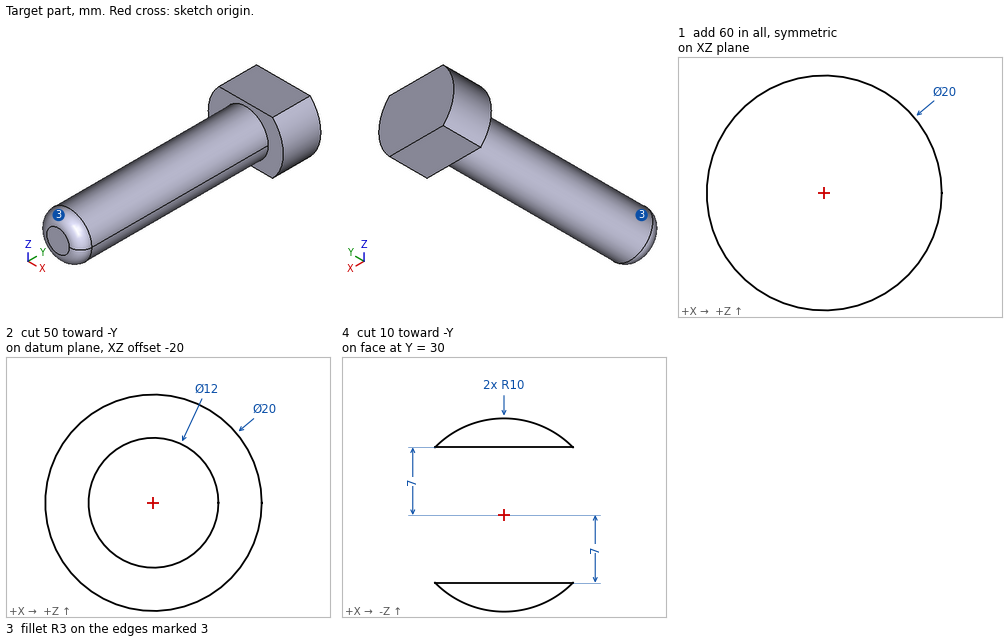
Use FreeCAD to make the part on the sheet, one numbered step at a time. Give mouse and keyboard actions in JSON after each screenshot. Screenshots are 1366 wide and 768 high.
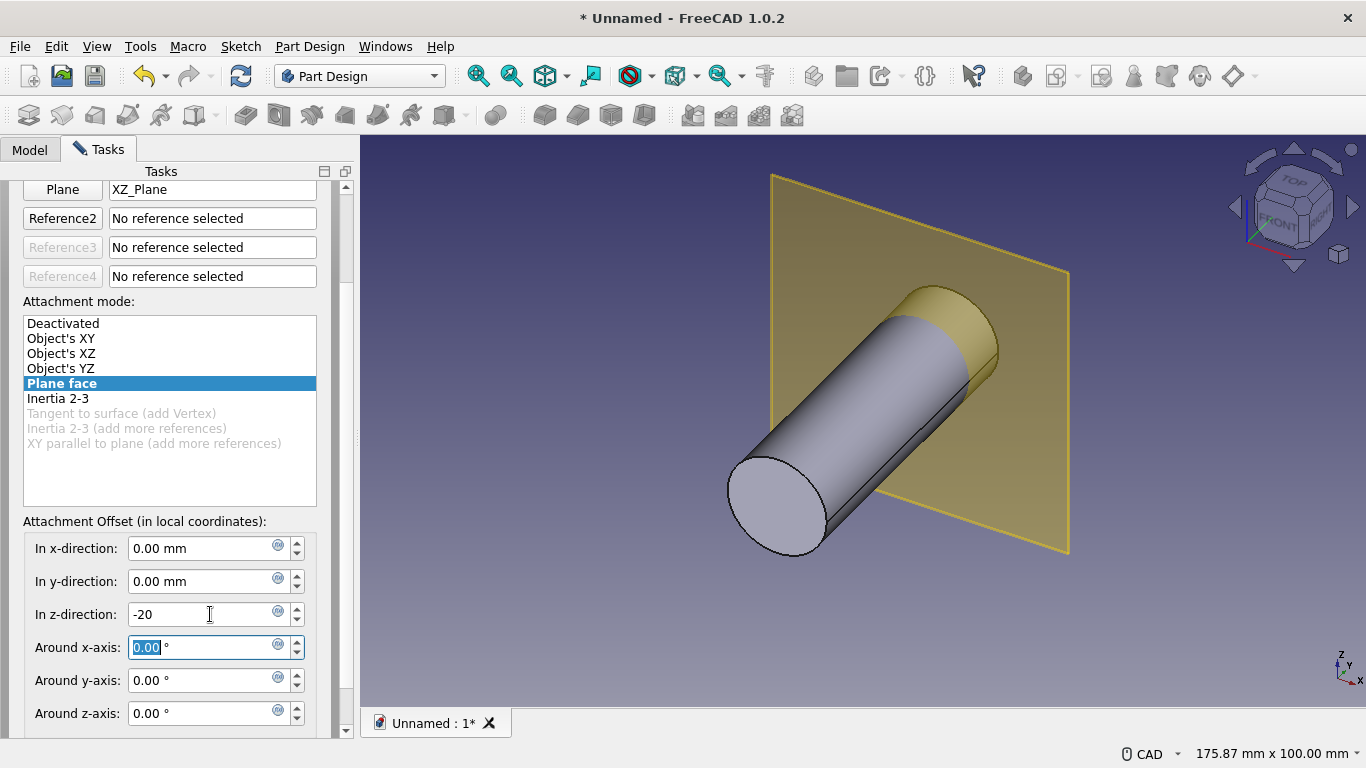
{"action": "scroll", "coordinate": [346, 460], "scroll_direction": "up", "scroll_amount": 3}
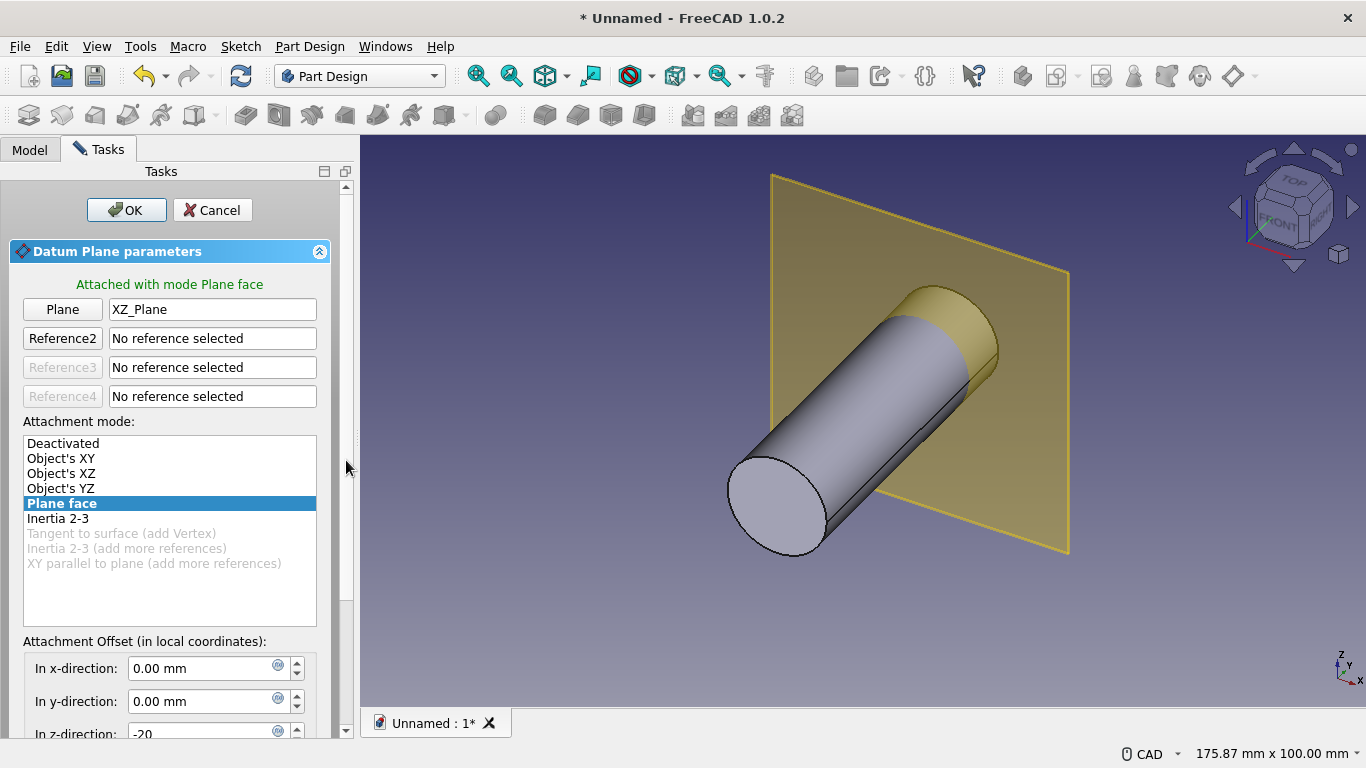
{"action": "left_click", "coordinate": [127, 210]}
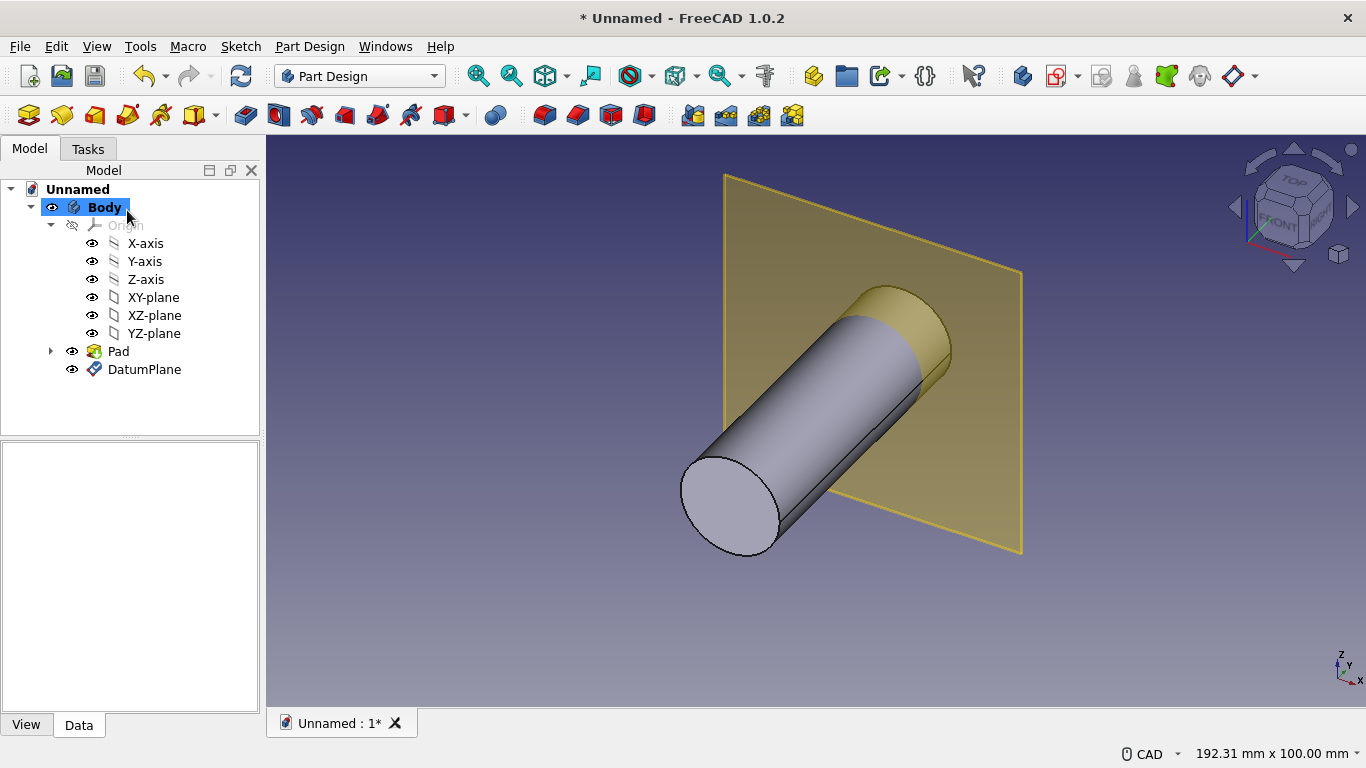
{"action": "left_click", "coordinate": [117, 369]}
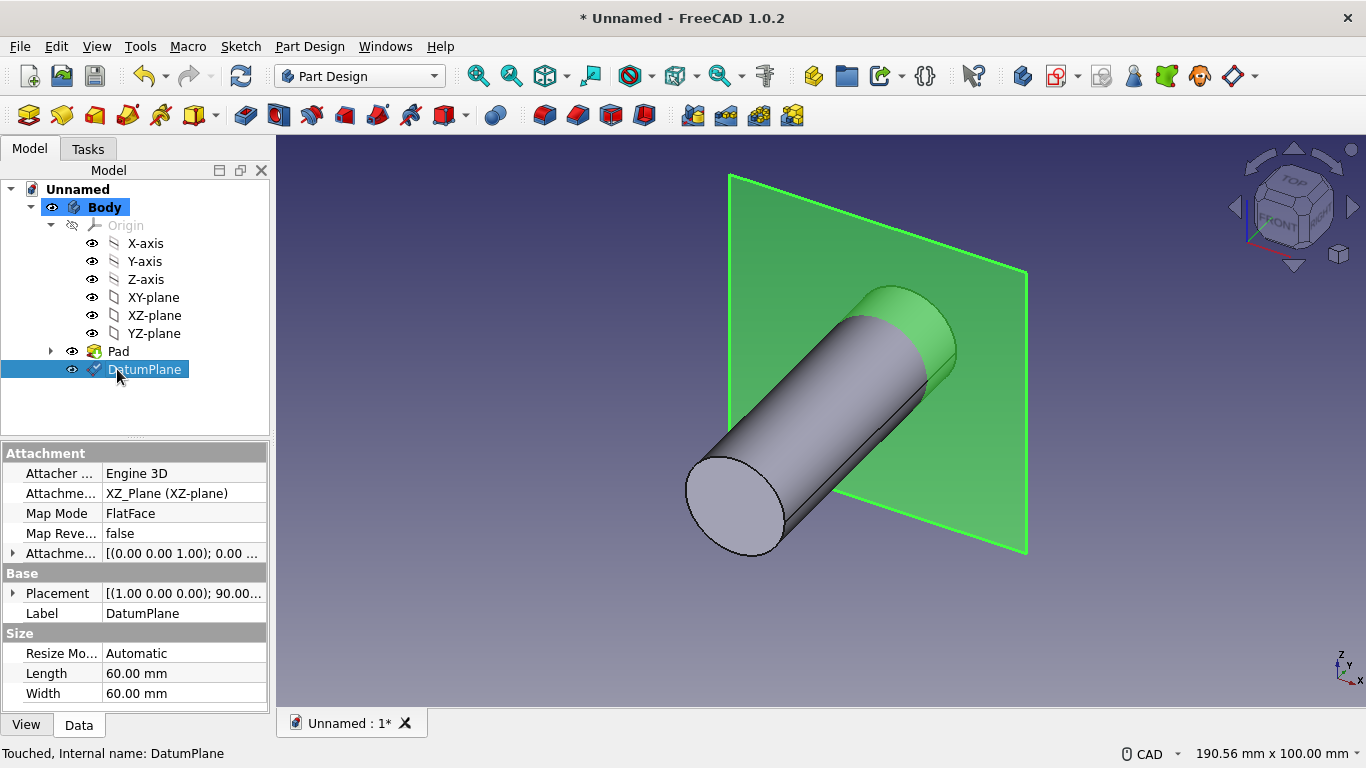
{"action": "left_click", "coordinate": [1056, 76]}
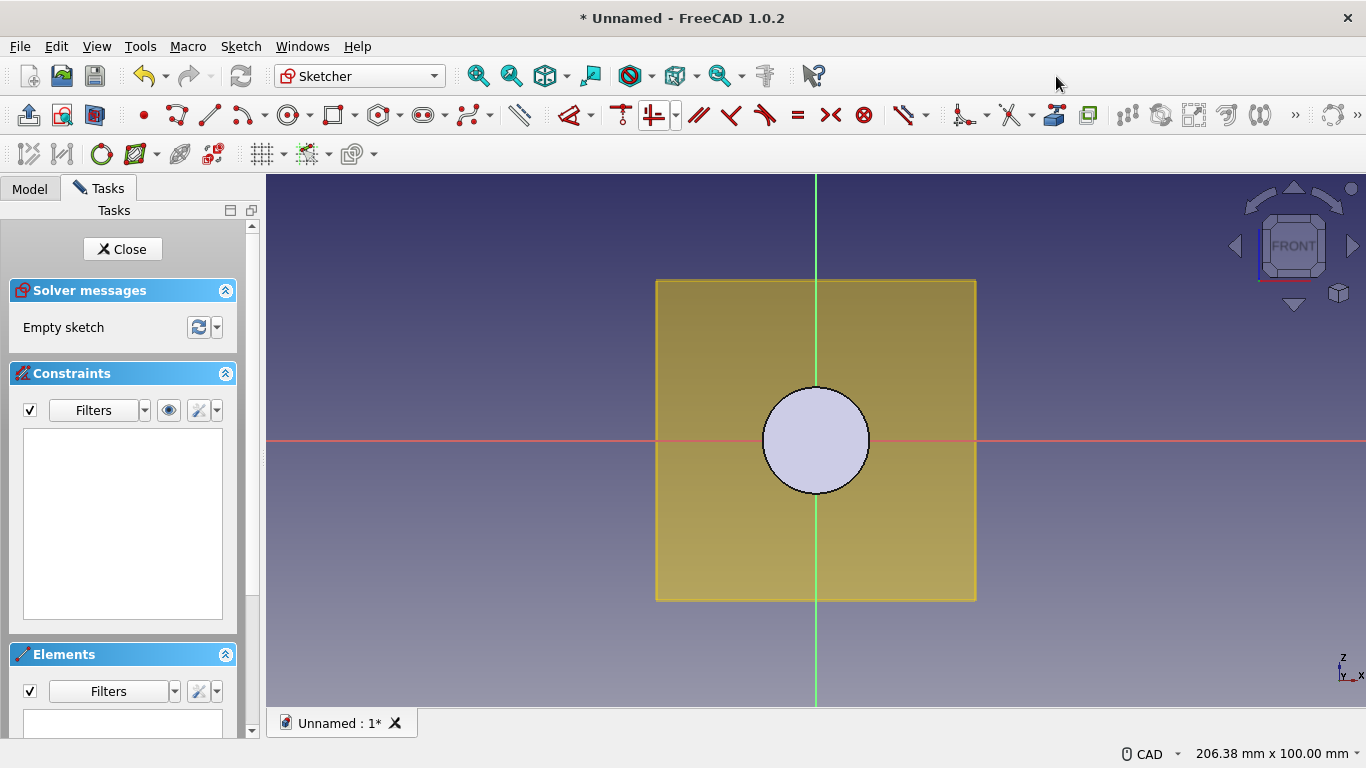
{"action": "left_click", "coordinate": [95, 116]}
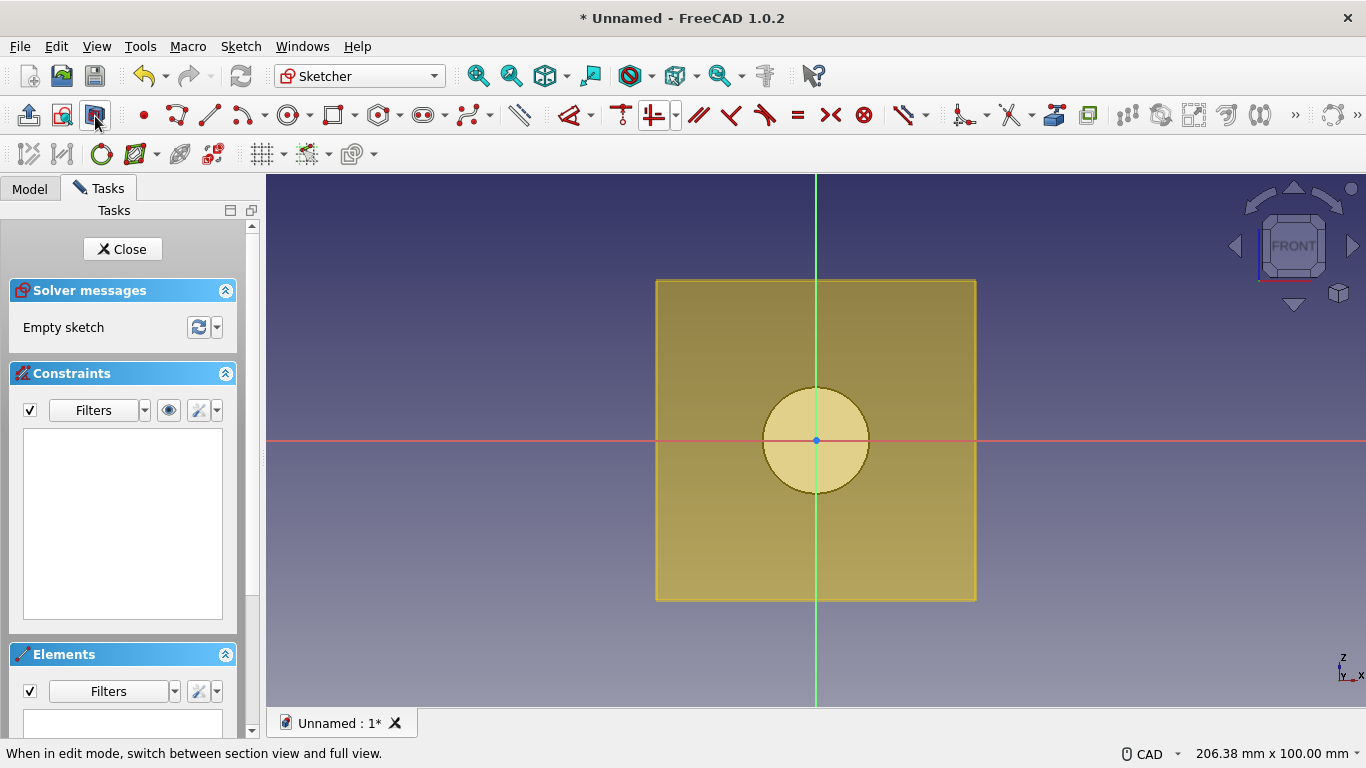
{"action": "scroll", "coordinate": [846, 440], "scroll_direction": "up", "scroll_amount": 6}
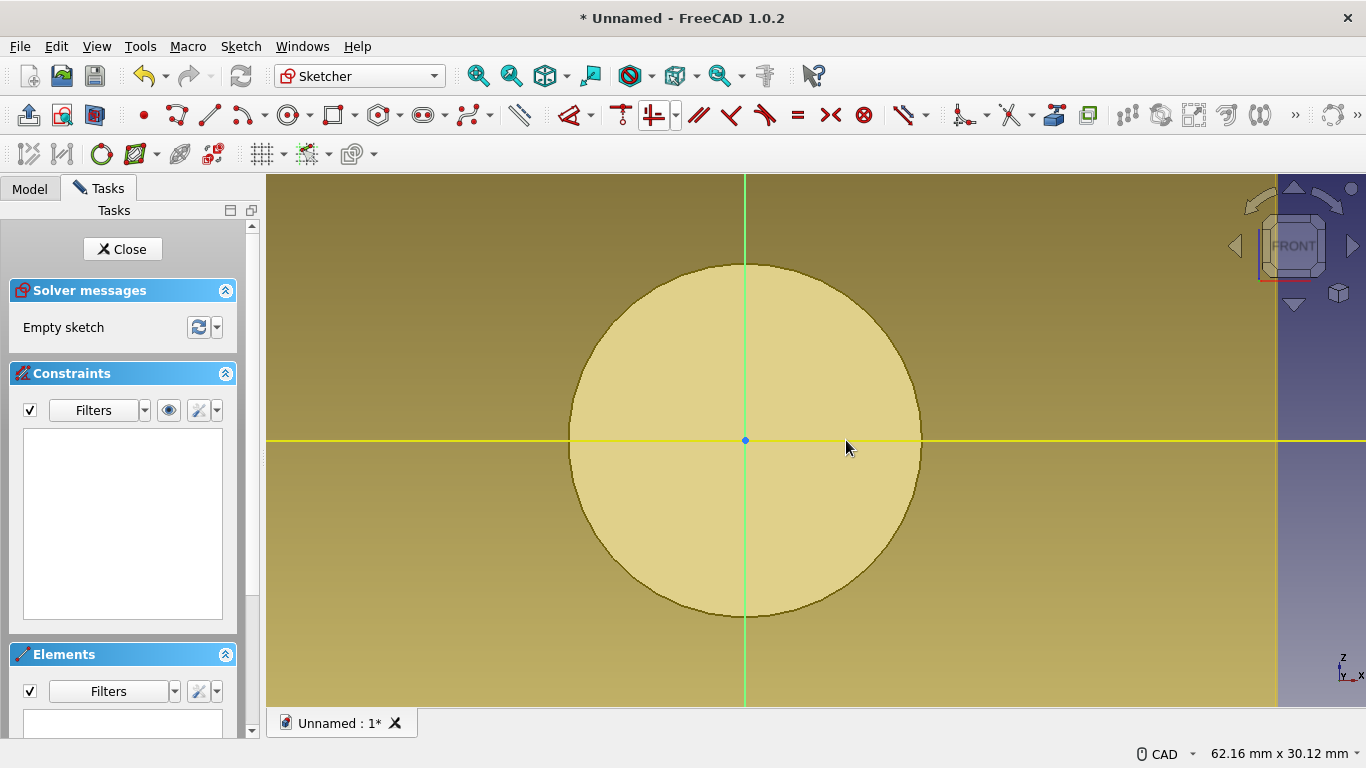
{"action": "left_click", "coordinate": [288, 116]}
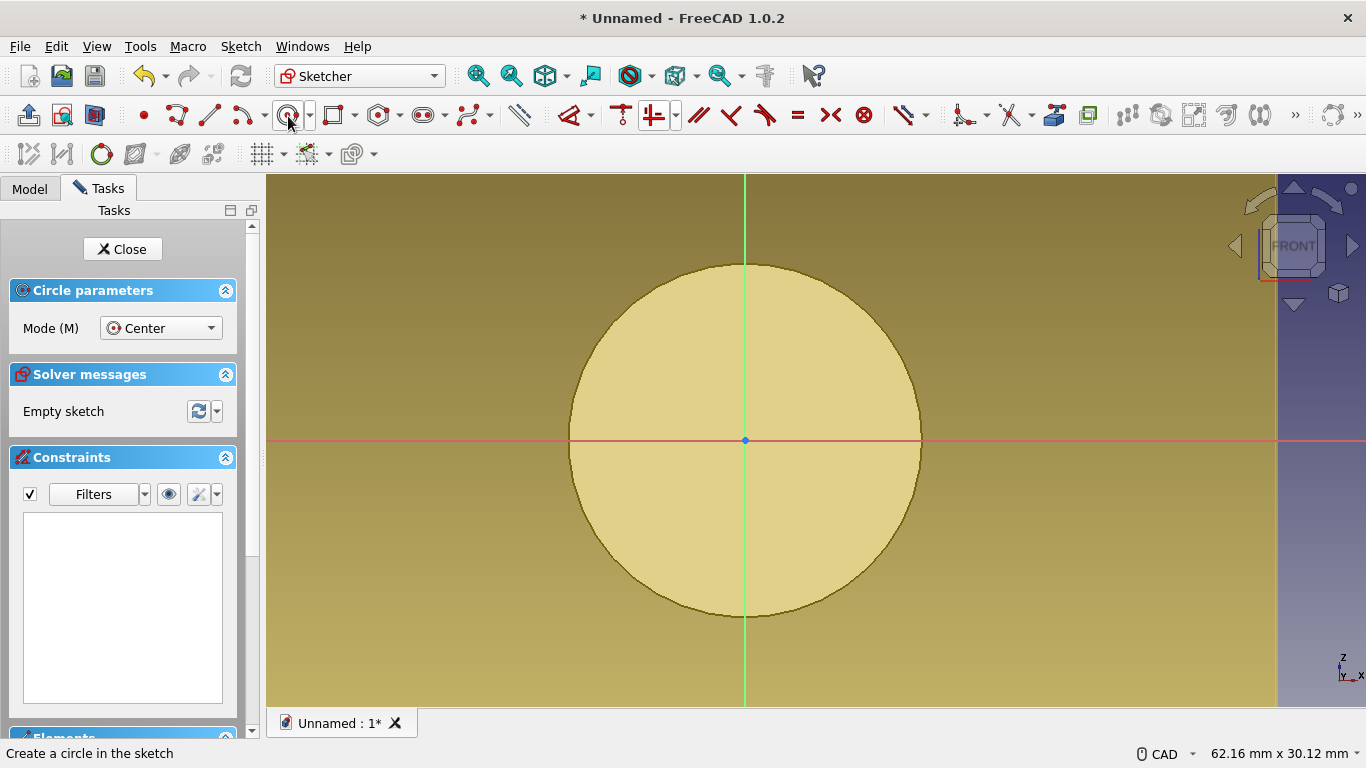
{"action": "left_click", "coordinate": [745, 441]}
{"action": "mouse_move", "coordinate": [870, 315]}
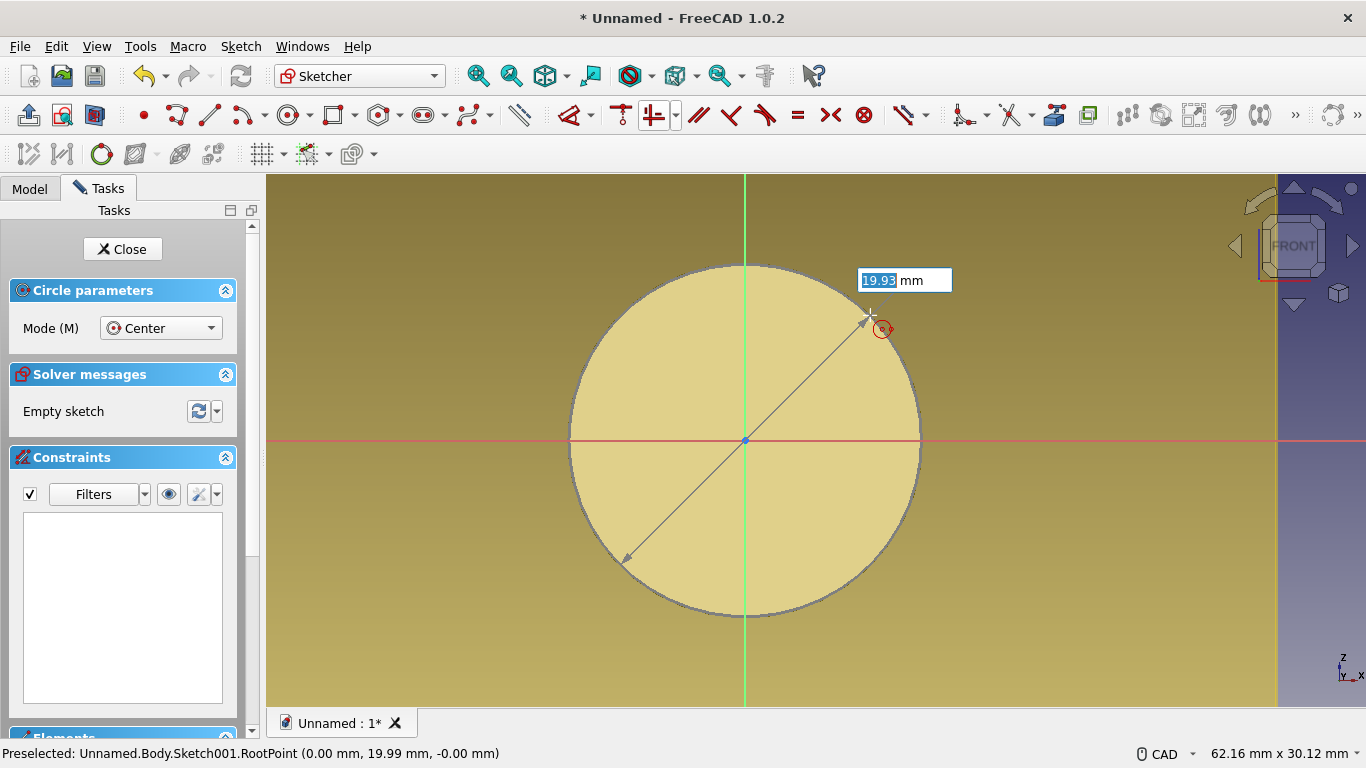
{"action": "type", "text": "20"}
{"action": "key", "text": "Return"}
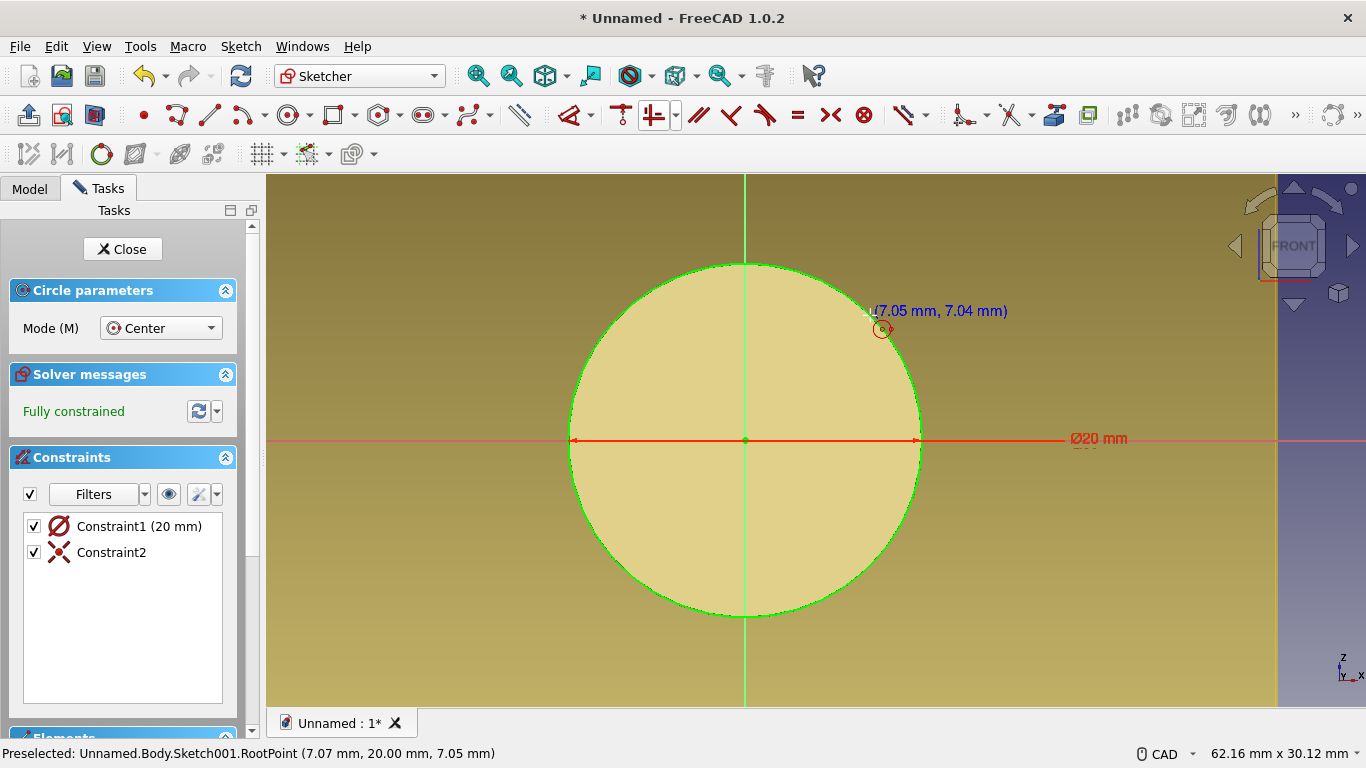
{"action": "left_click", "coordinate": [745, 441]}
{"action": "mouse_move", "coordinate": [820, 365]}